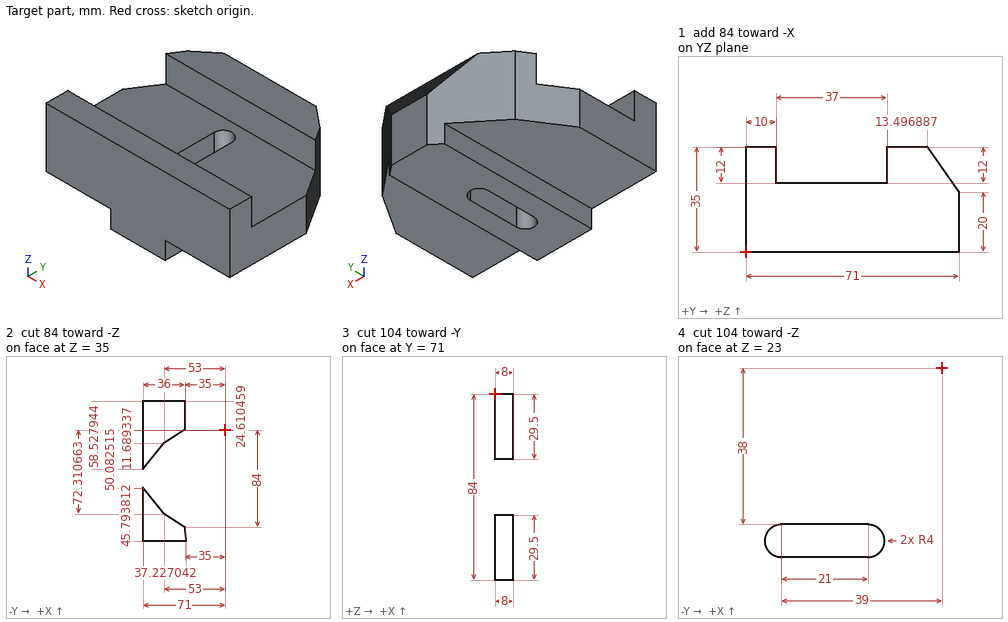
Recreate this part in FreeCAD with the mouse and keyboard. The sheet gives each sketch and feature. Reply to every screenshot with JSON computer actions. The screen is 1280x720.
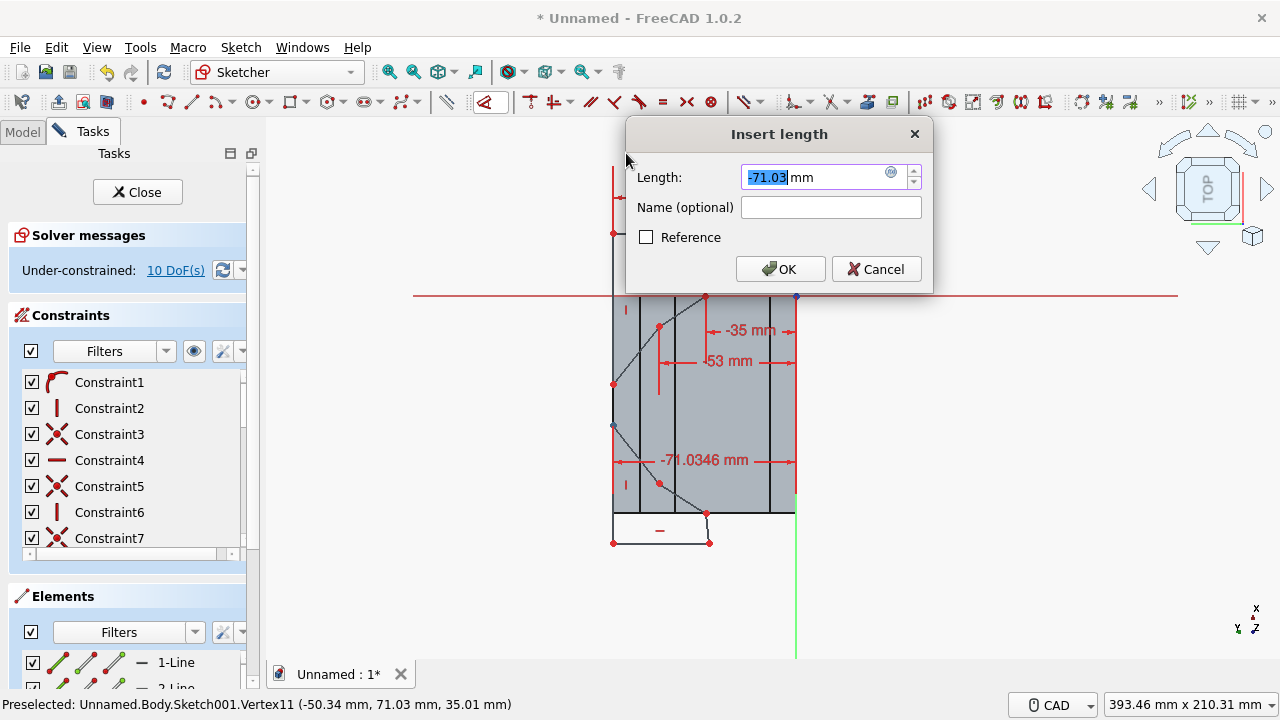
{"action": "type", "text": "-71"}
{"action": "key", "text": "Return"}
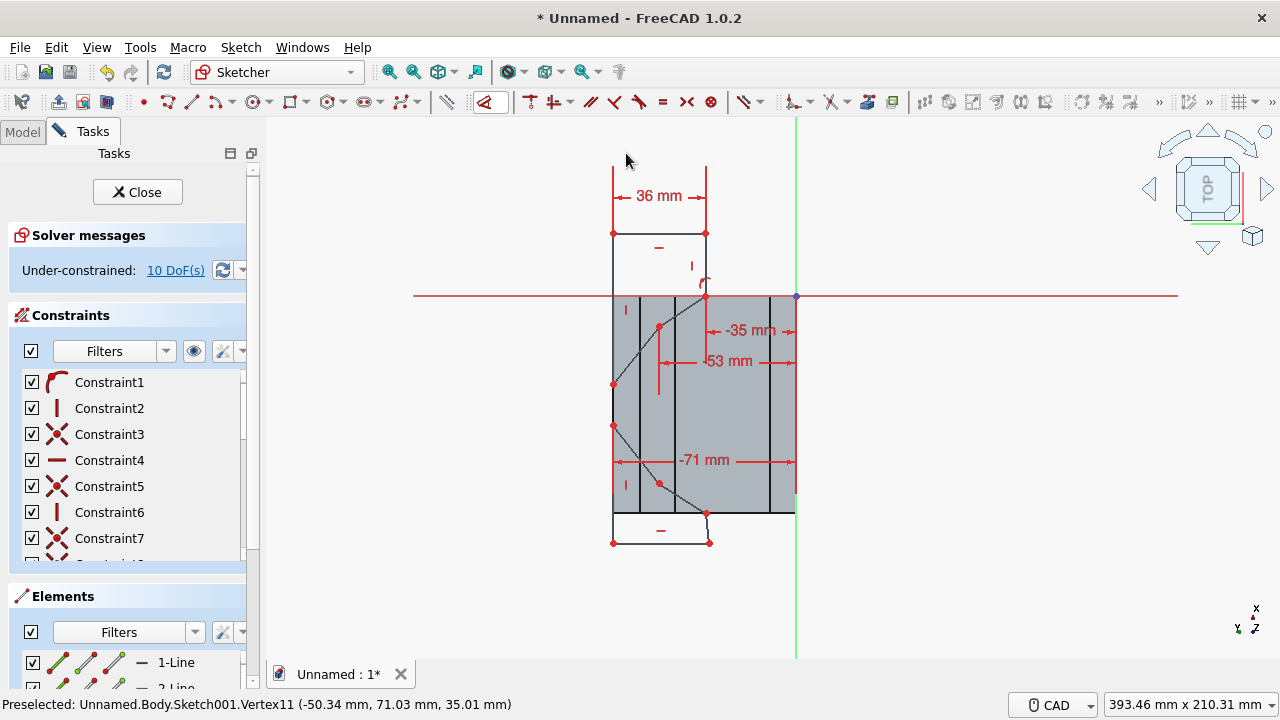
{"action": "left_click", "coordinate": [706, 514]}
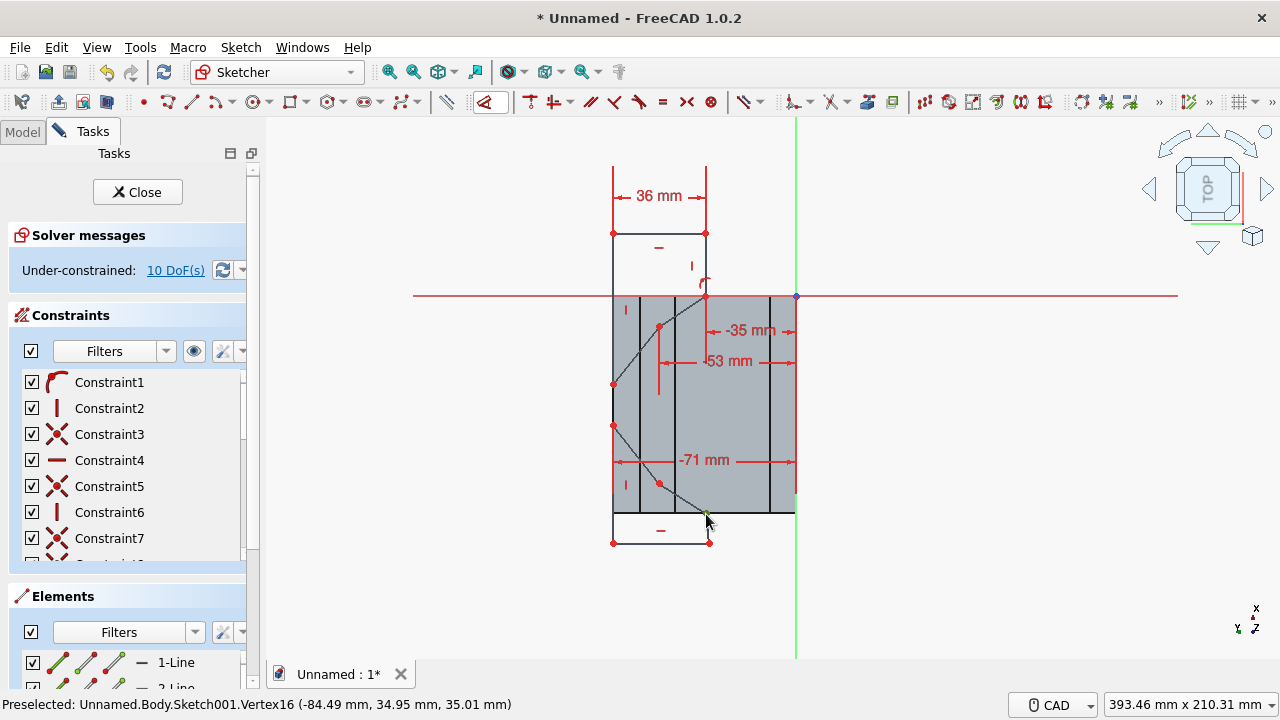
{"action": "key", "text": "l"}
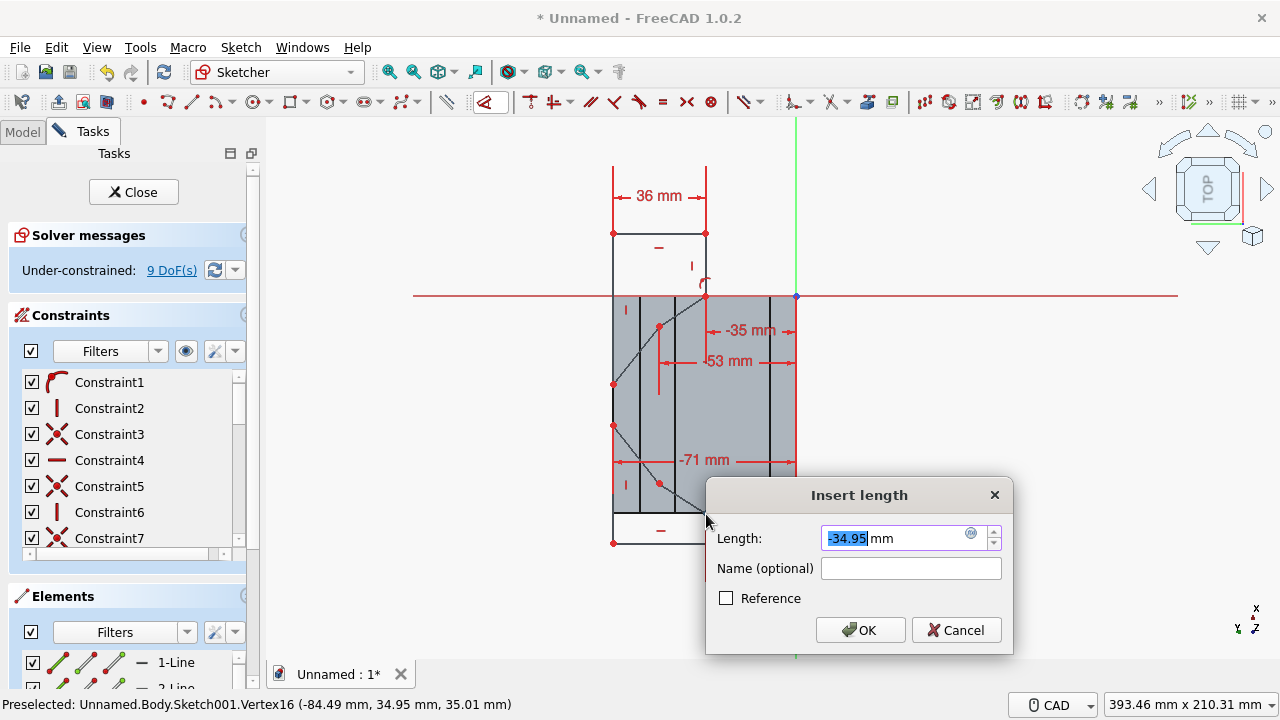
{"action": "type", "text": "-35"}
{"action": "key", "text": "Return"}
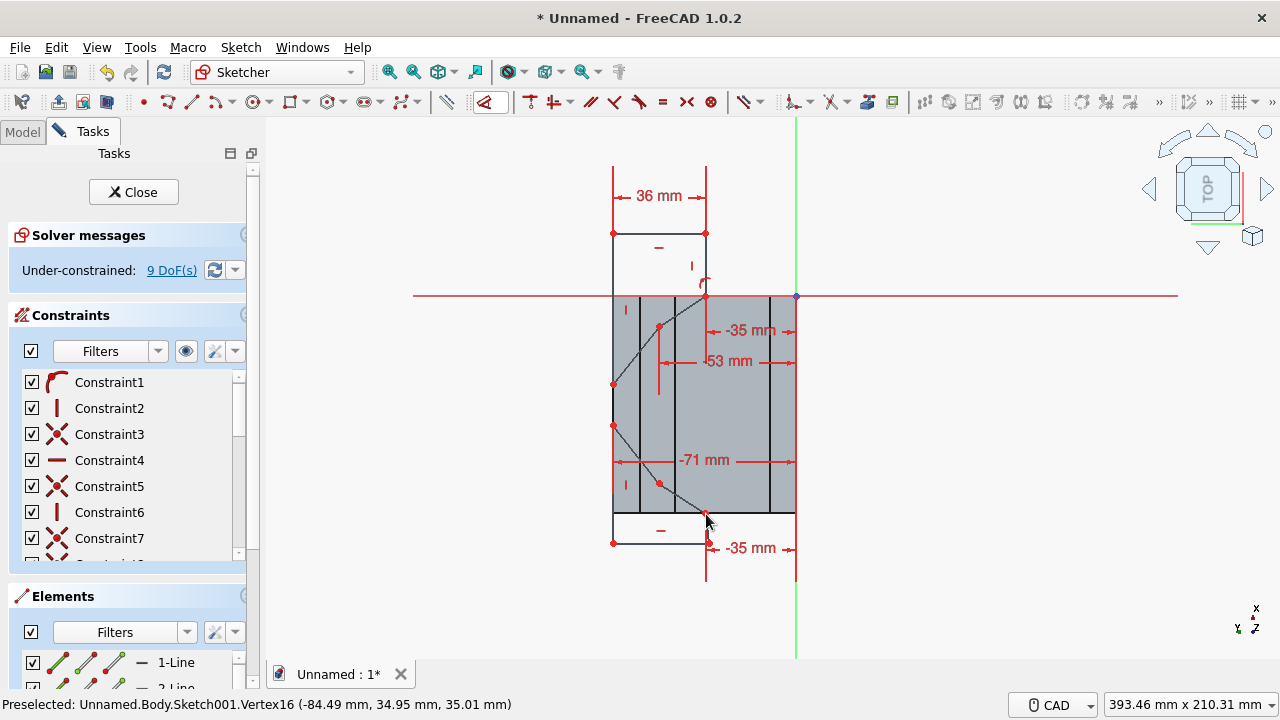
{"action": "left_click", "coordinate": [706, 514]}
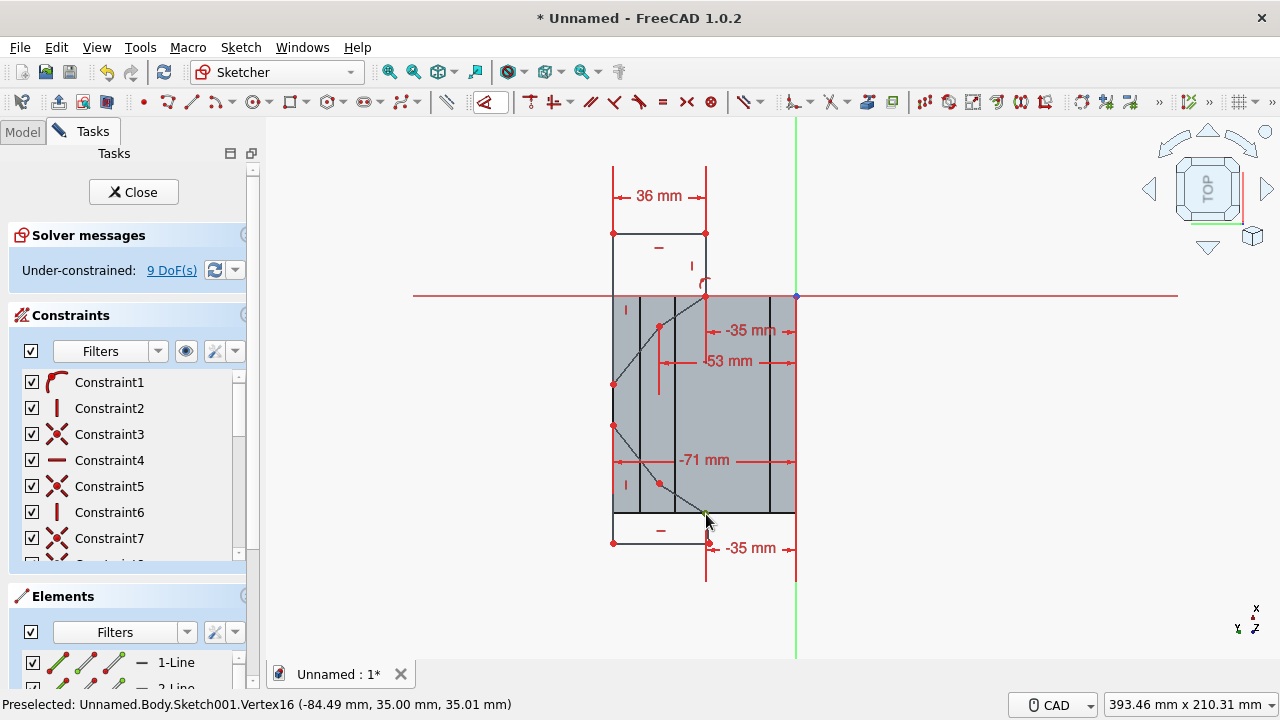
{"action": "key", "text": "i"}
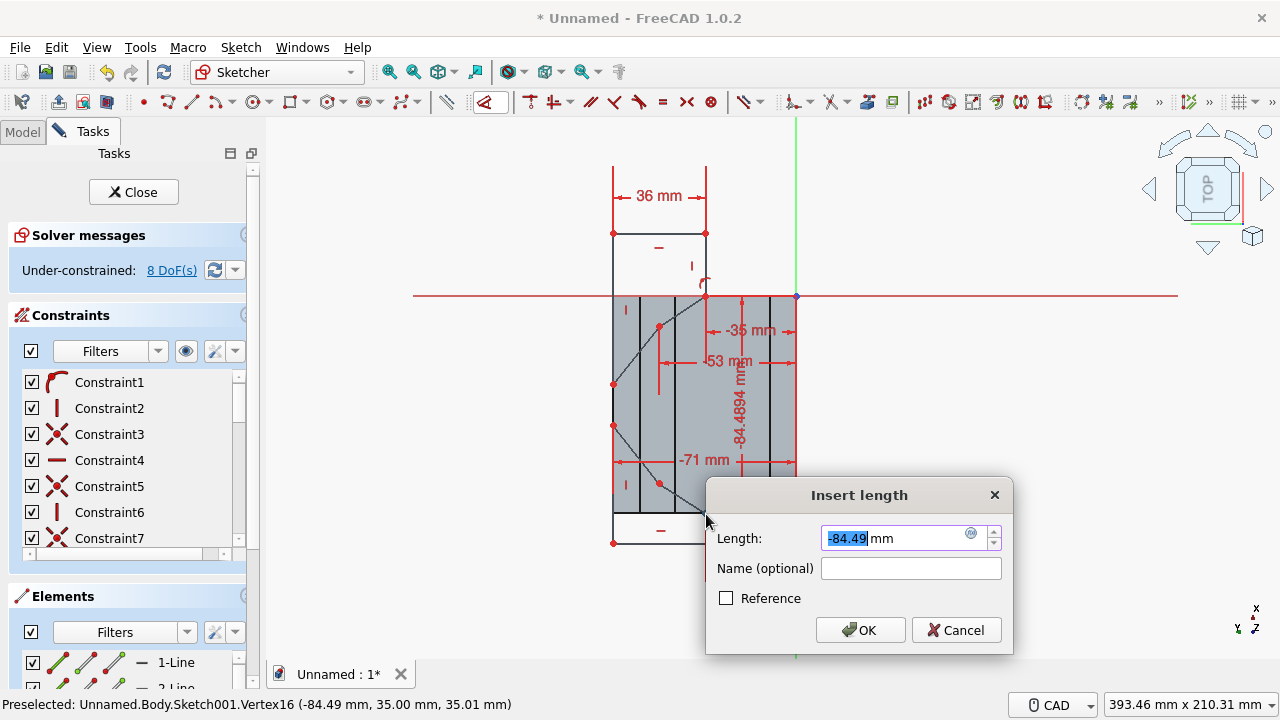
{"action": "type", "text": "-84"}
{"action": "key", "text": "Return"}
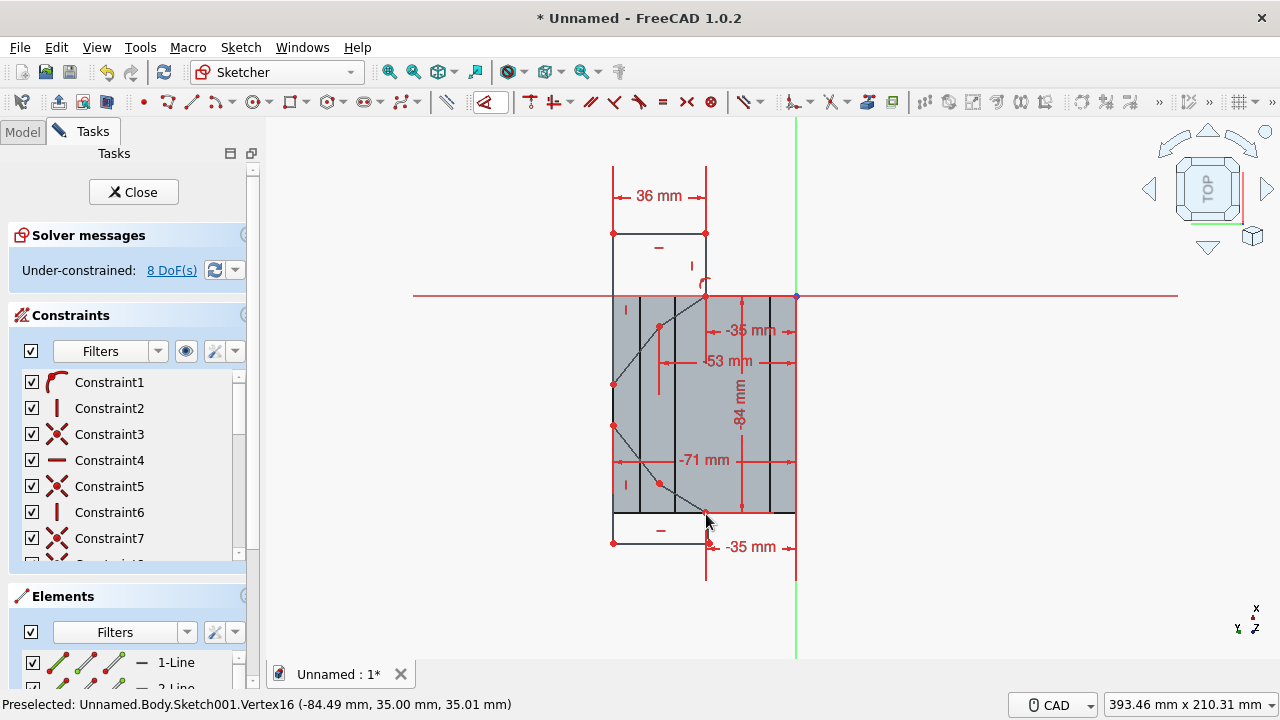
{"action": "left_click", "coordinate": [659, 484]}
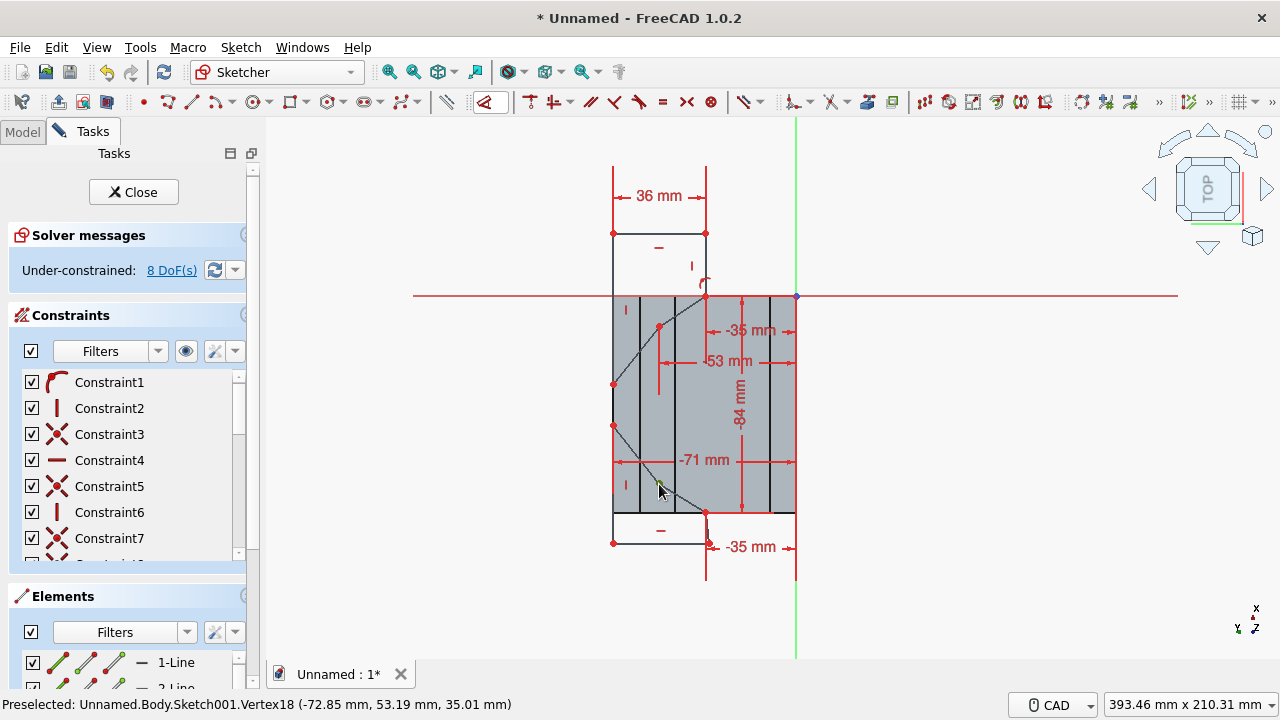
{"action": "key", "text": "l"}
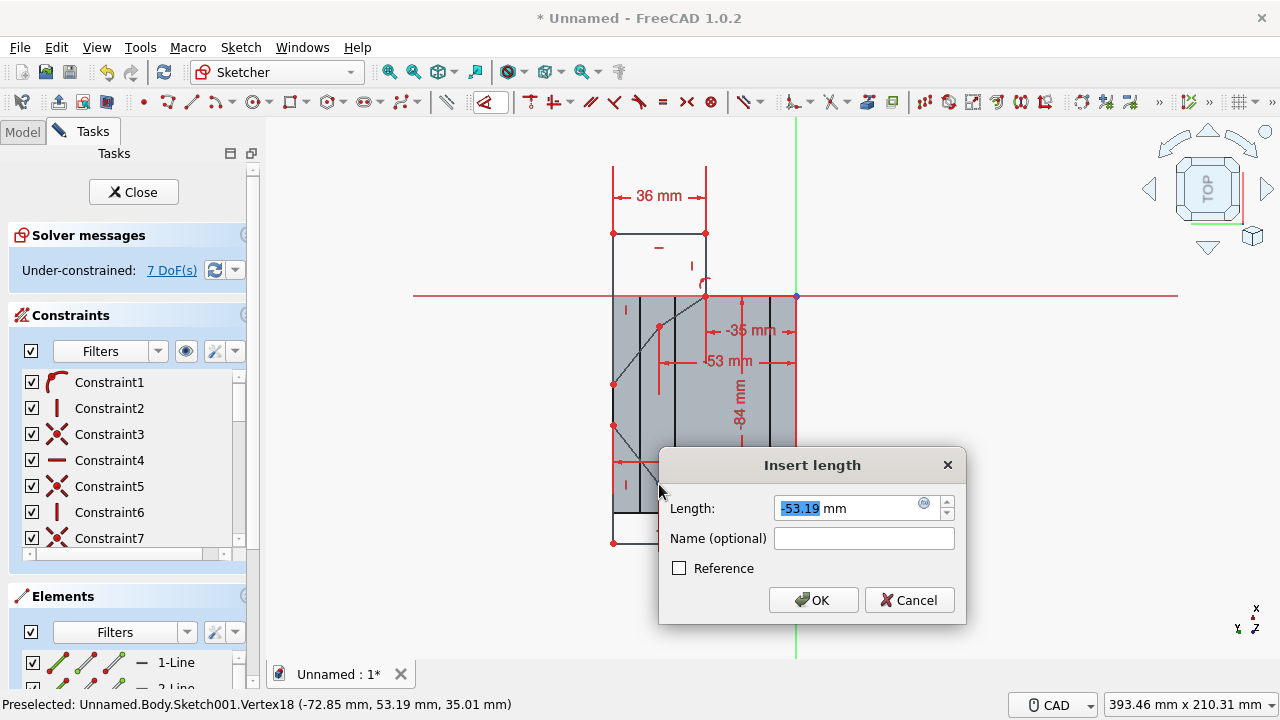
{"action": "type", "text": "-53"}
{"action": "key", "text": "Return"}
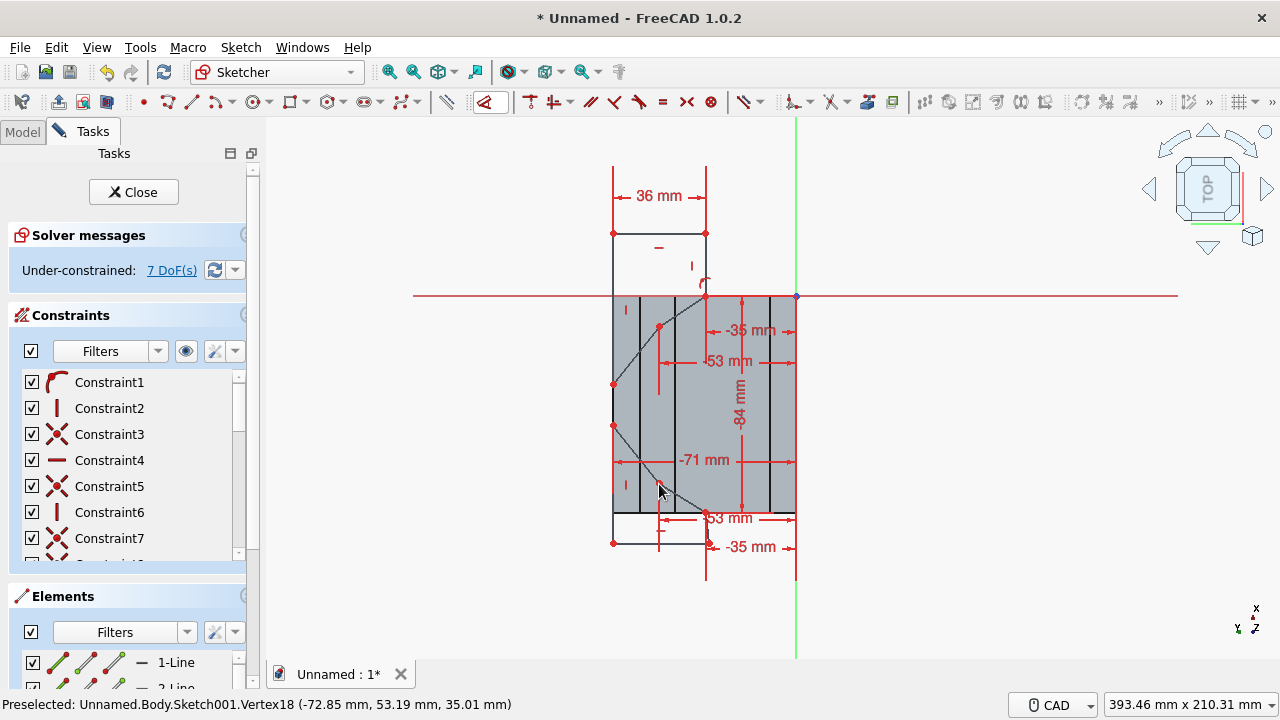
{"action": "left_click", "coordinate": [706, 253]}